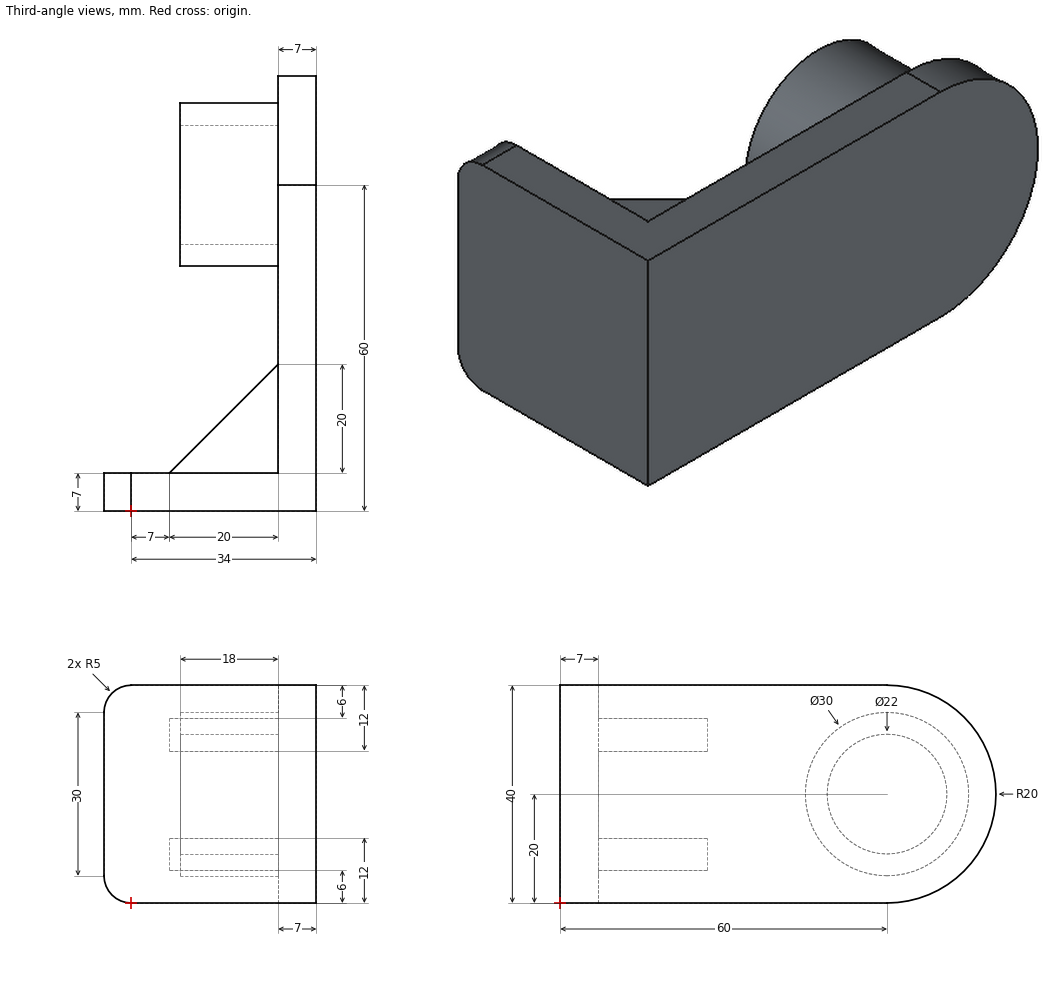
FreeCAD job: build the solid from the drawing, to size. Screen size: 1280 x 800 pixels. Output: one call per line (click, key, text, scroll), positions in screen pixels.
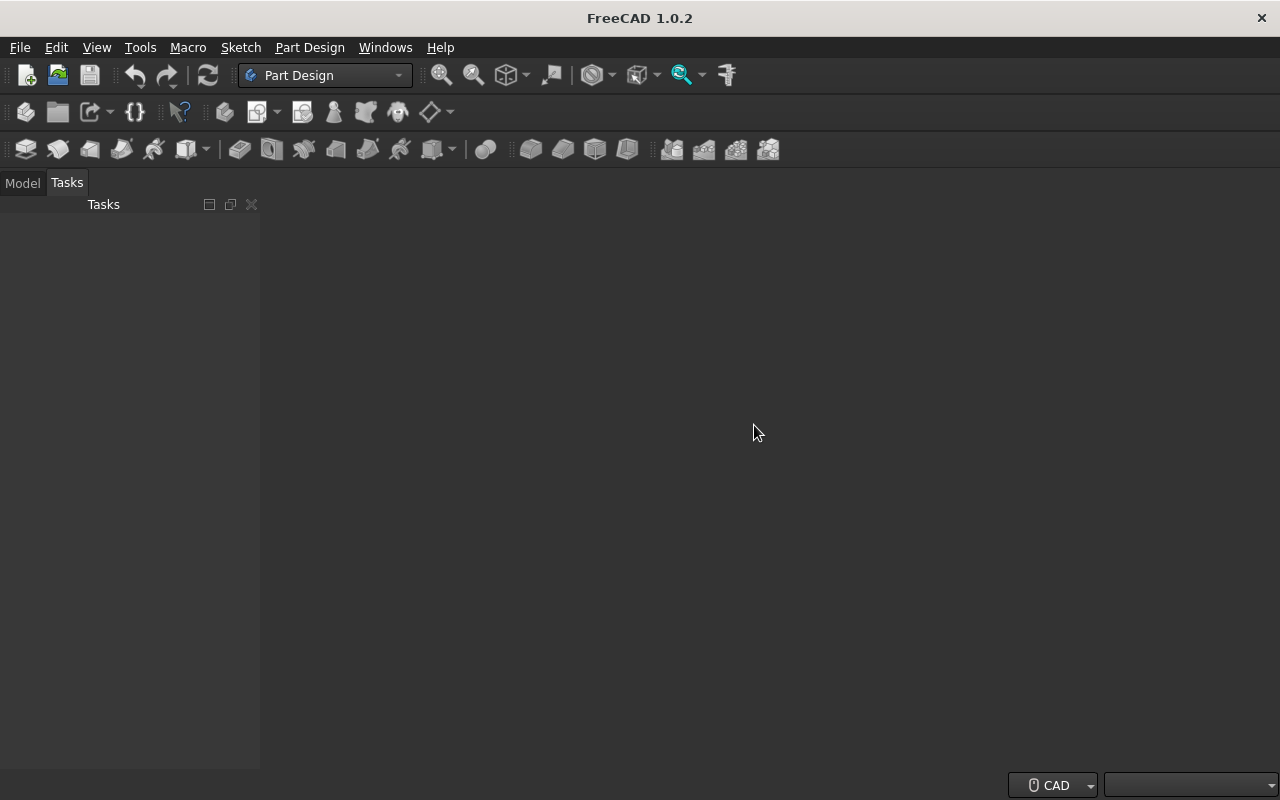
click(26, 76)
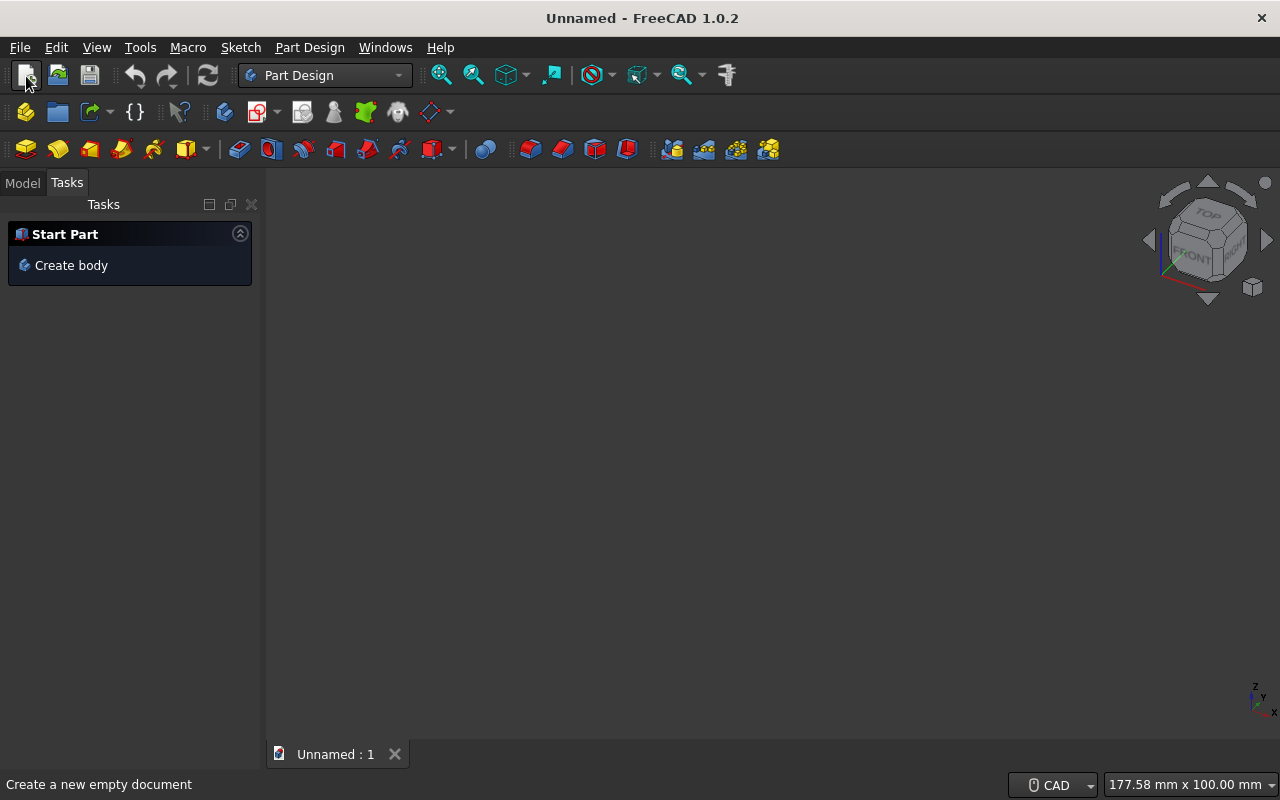
click(258, 112)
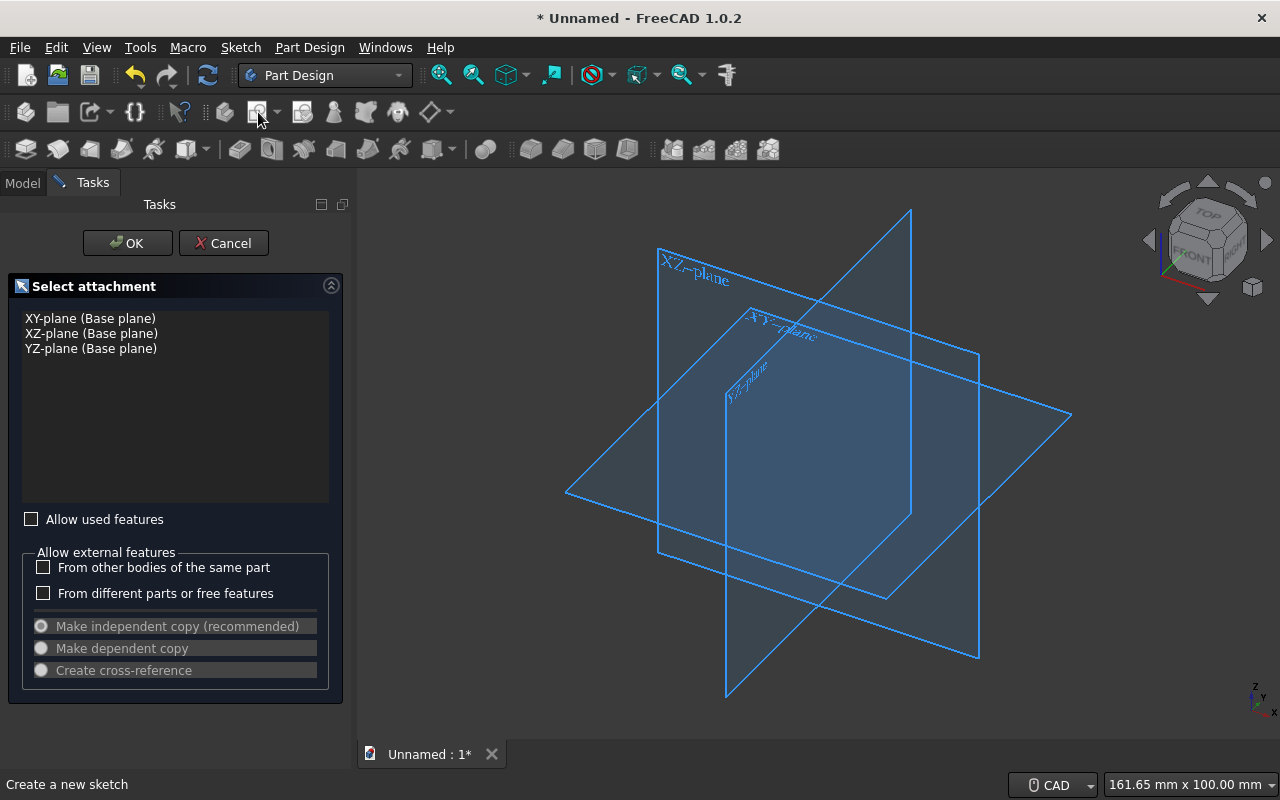
click(82, 318)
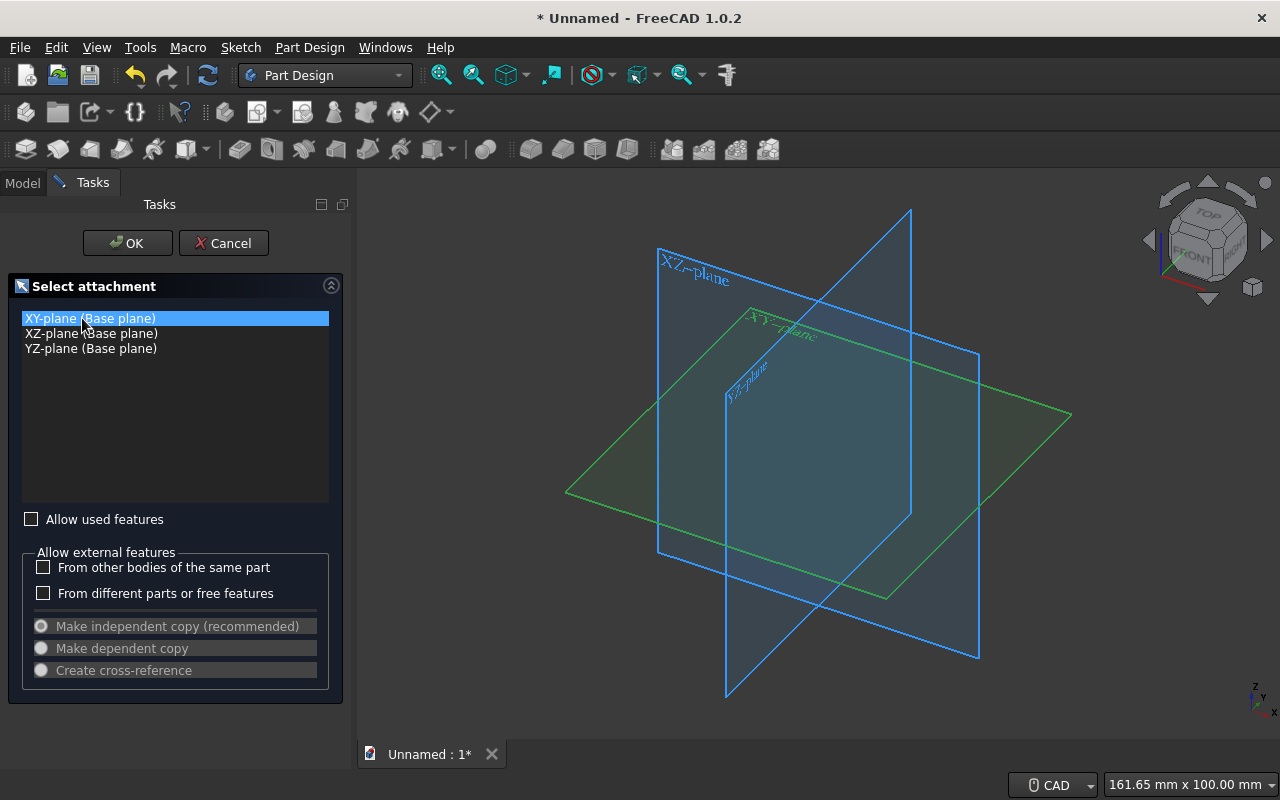
click(128, 243)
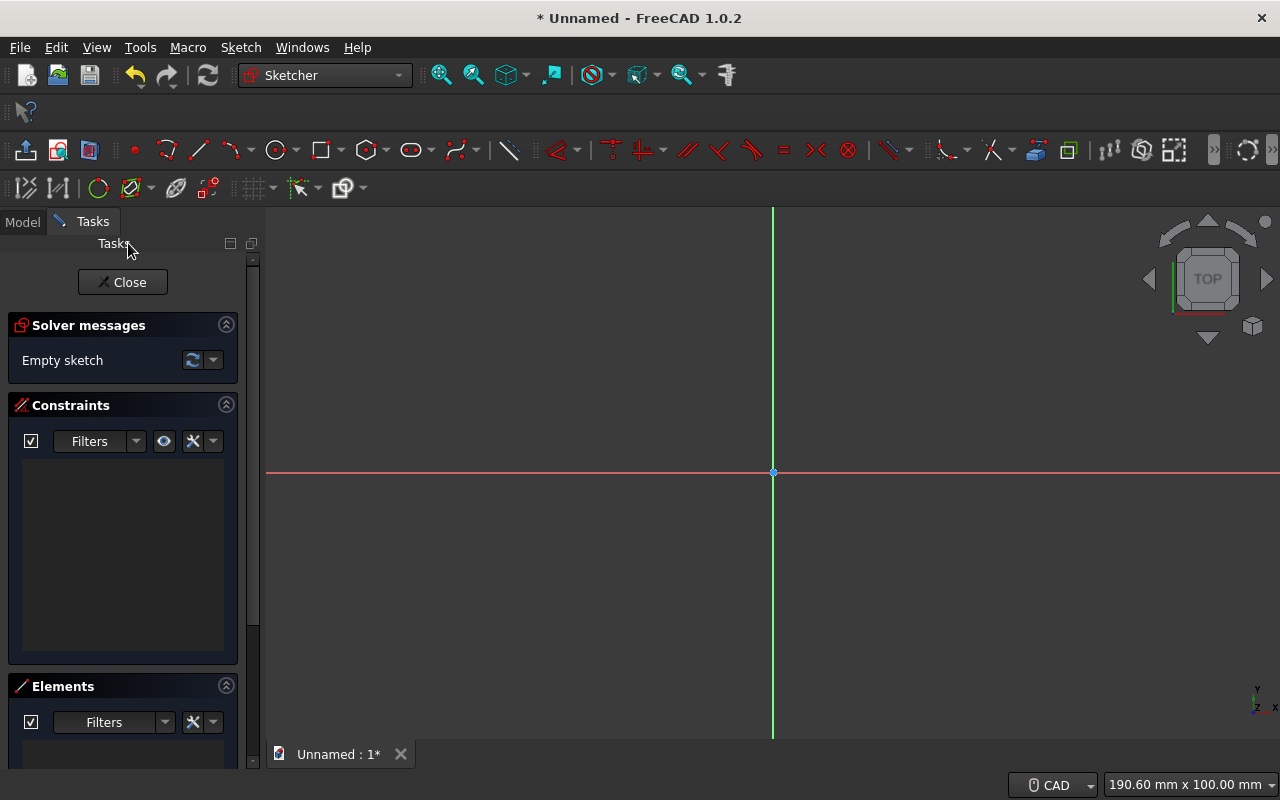
scroll(381, 711, down, 2)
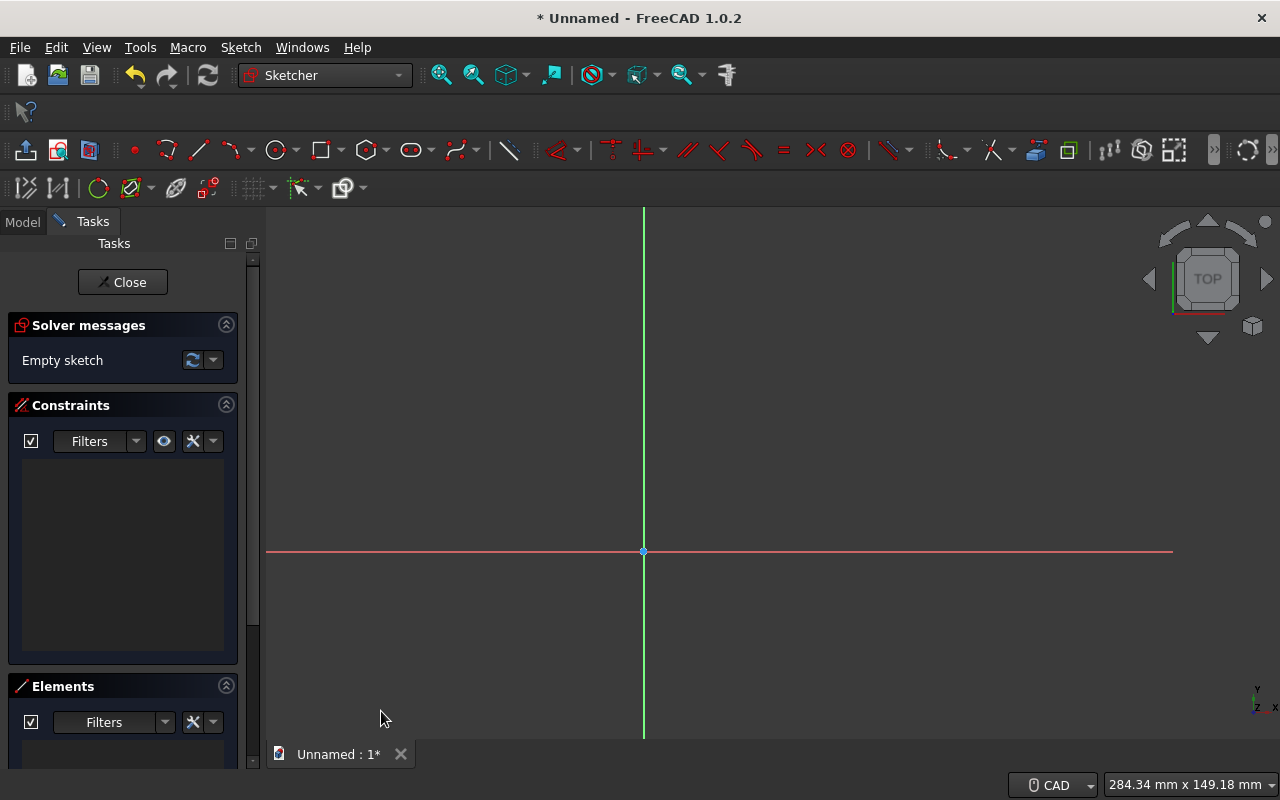
scroll(704, 387, up, 2)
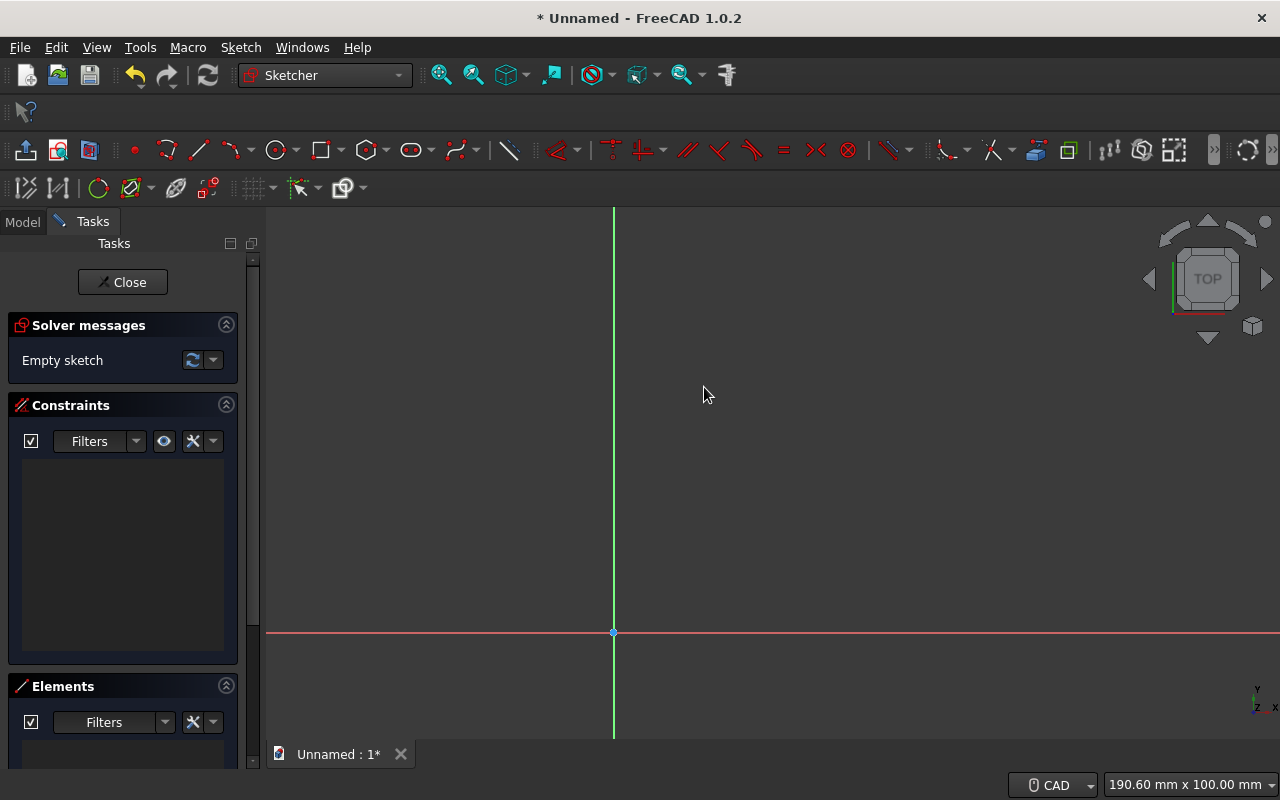
click(168, 150)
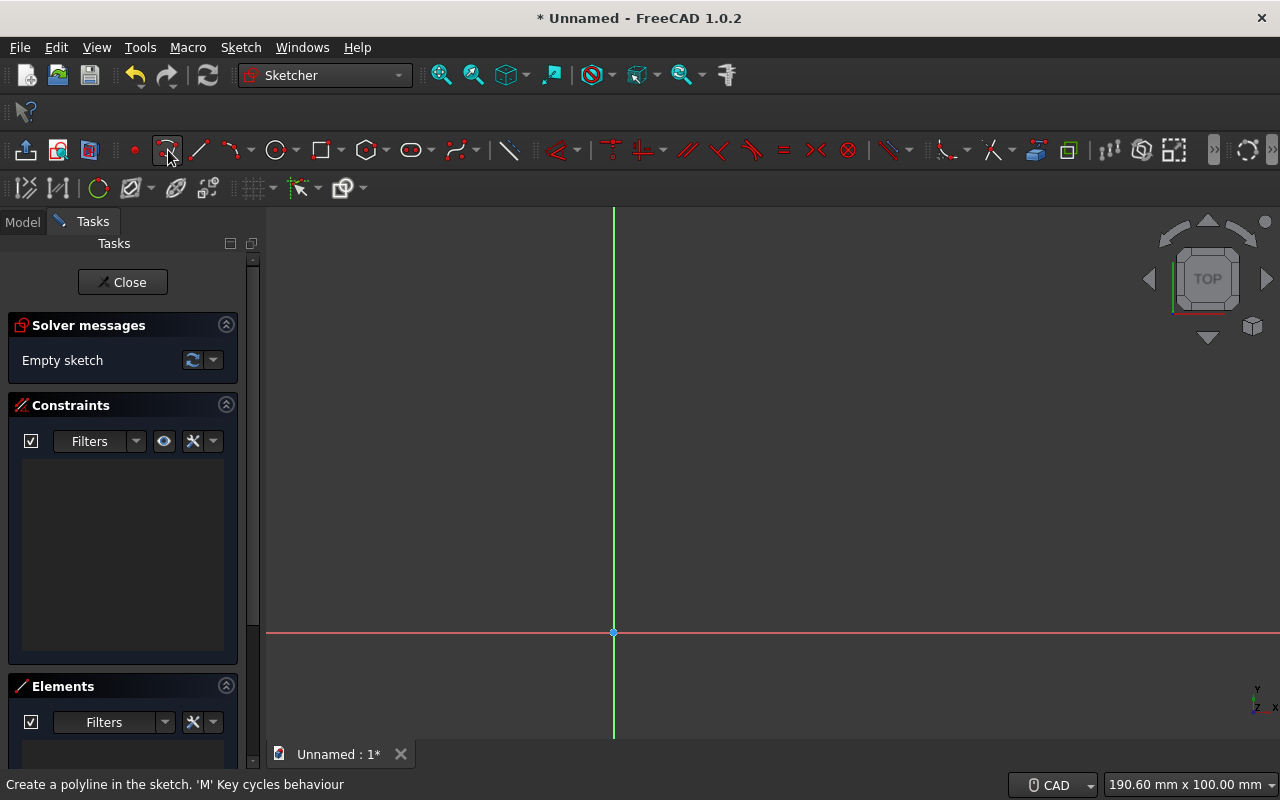
click(614, 633)
click(795, 624)
click(795, 313)
click(758, 313)
click(758, 595)
click(623, 595)
click(614, 633)
key(Escape)
key(Escape)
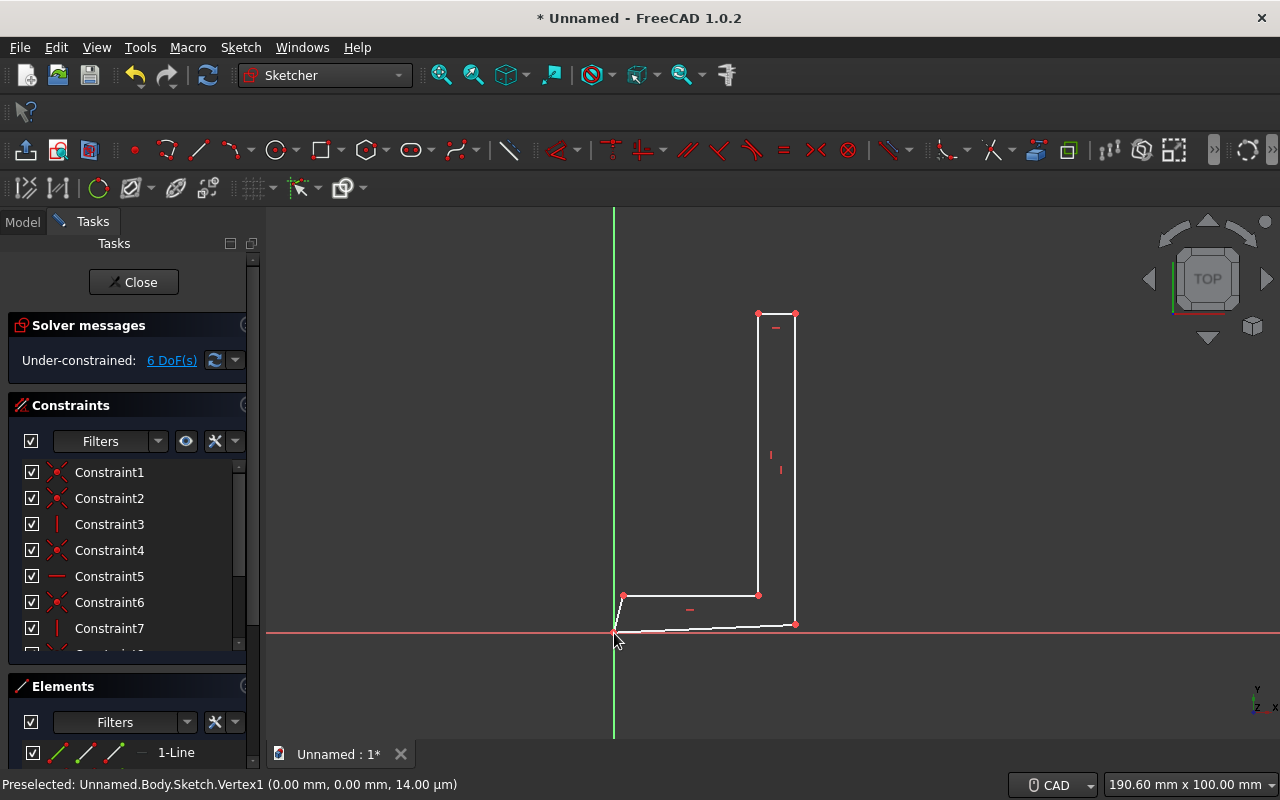
click(668, 630)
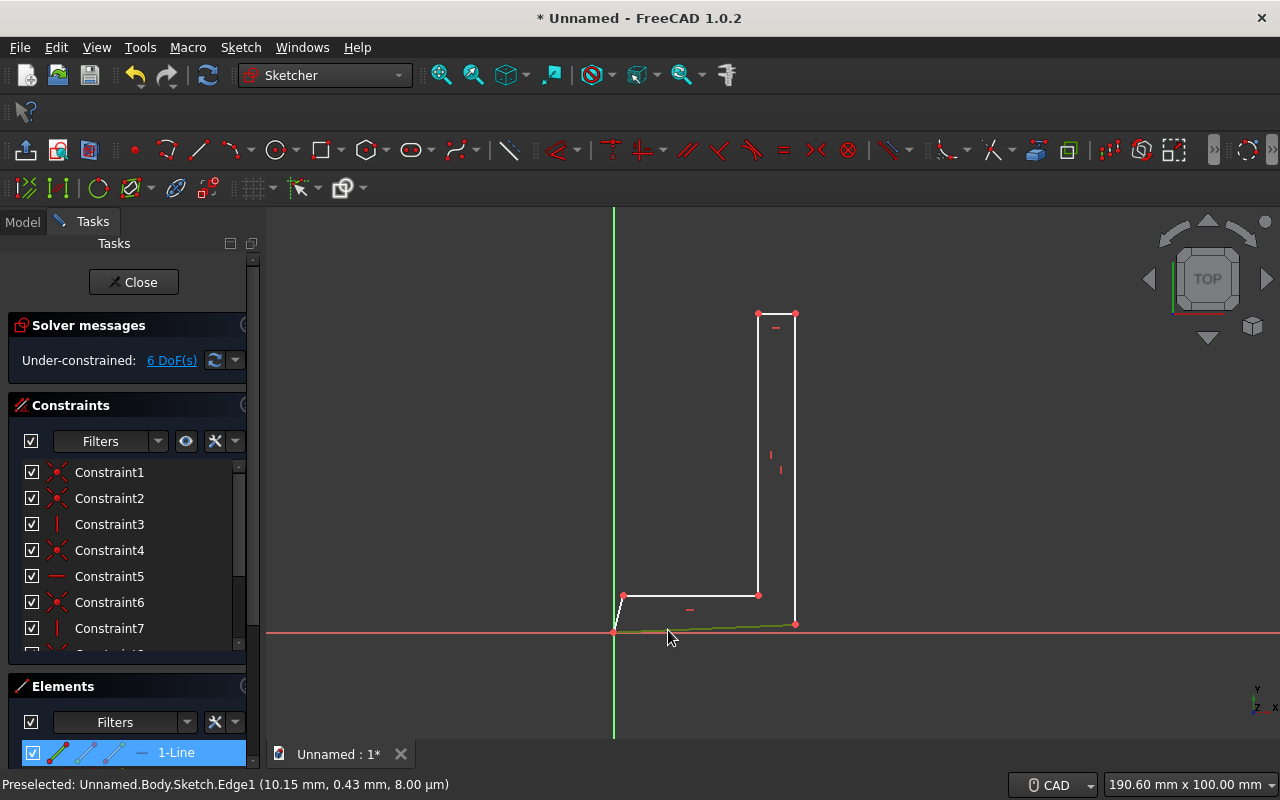
click(666, 150)